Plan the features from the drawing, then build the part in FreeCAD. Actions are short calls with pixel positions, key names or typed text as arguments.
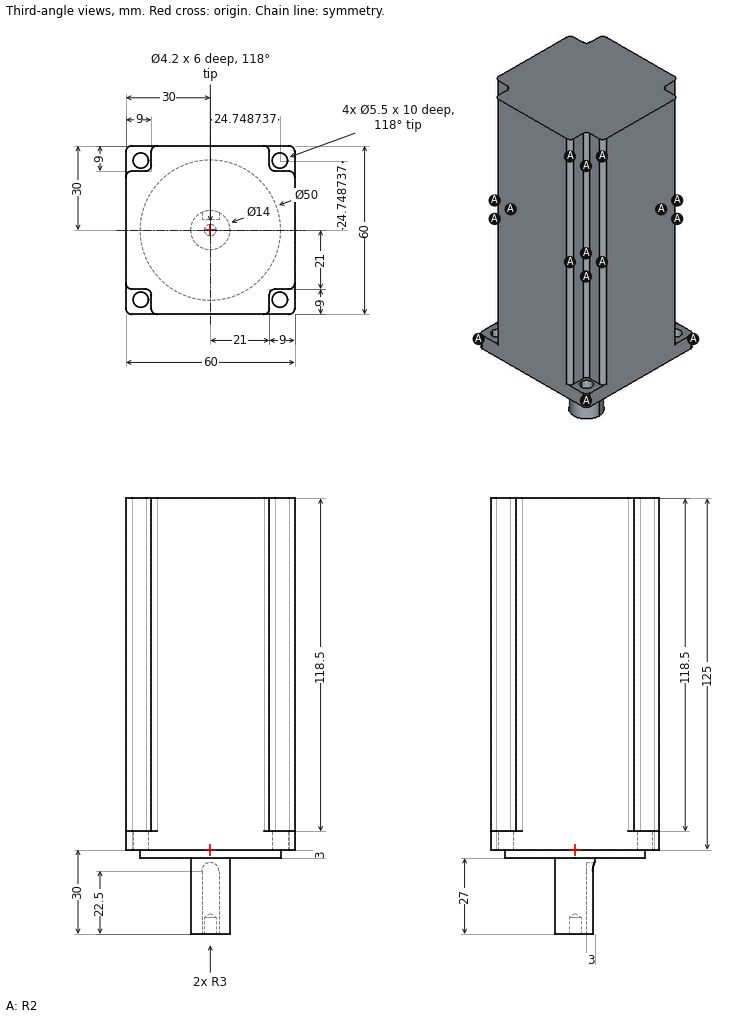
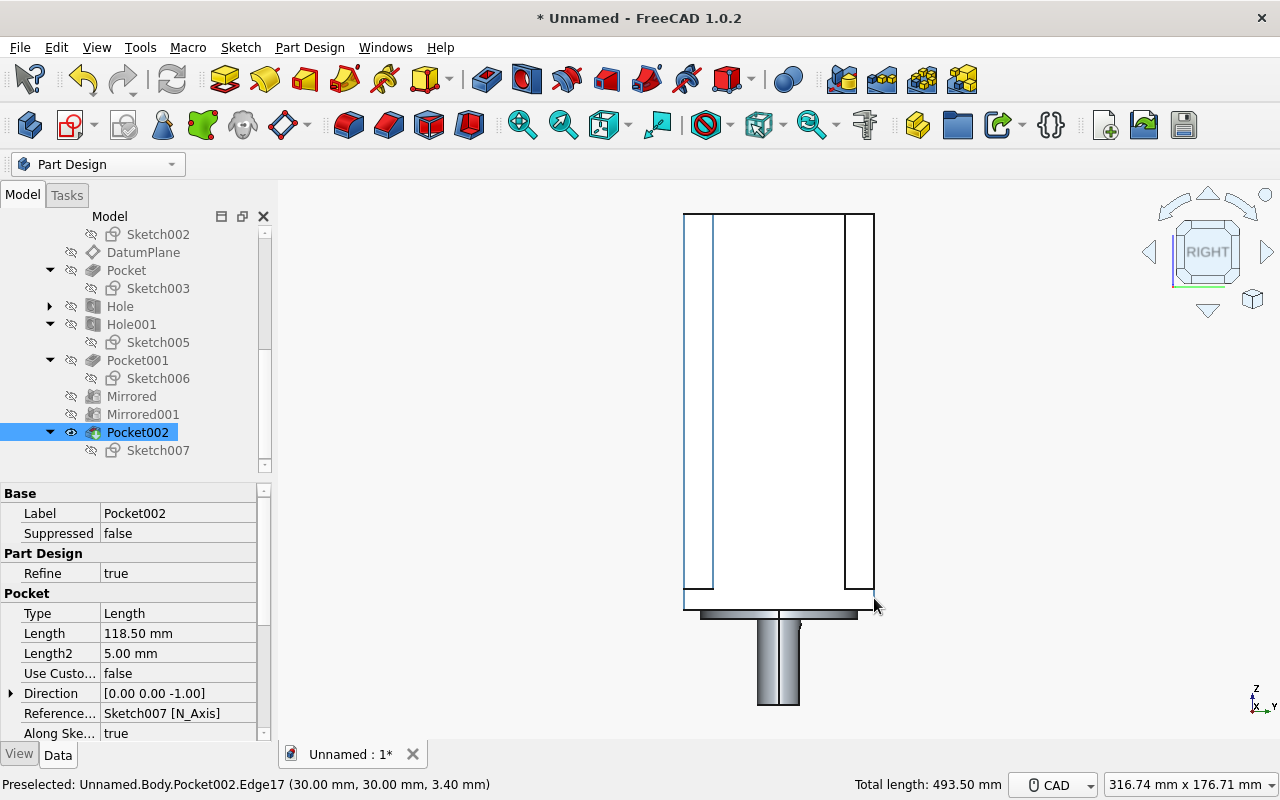
click(845, 401, ctrl)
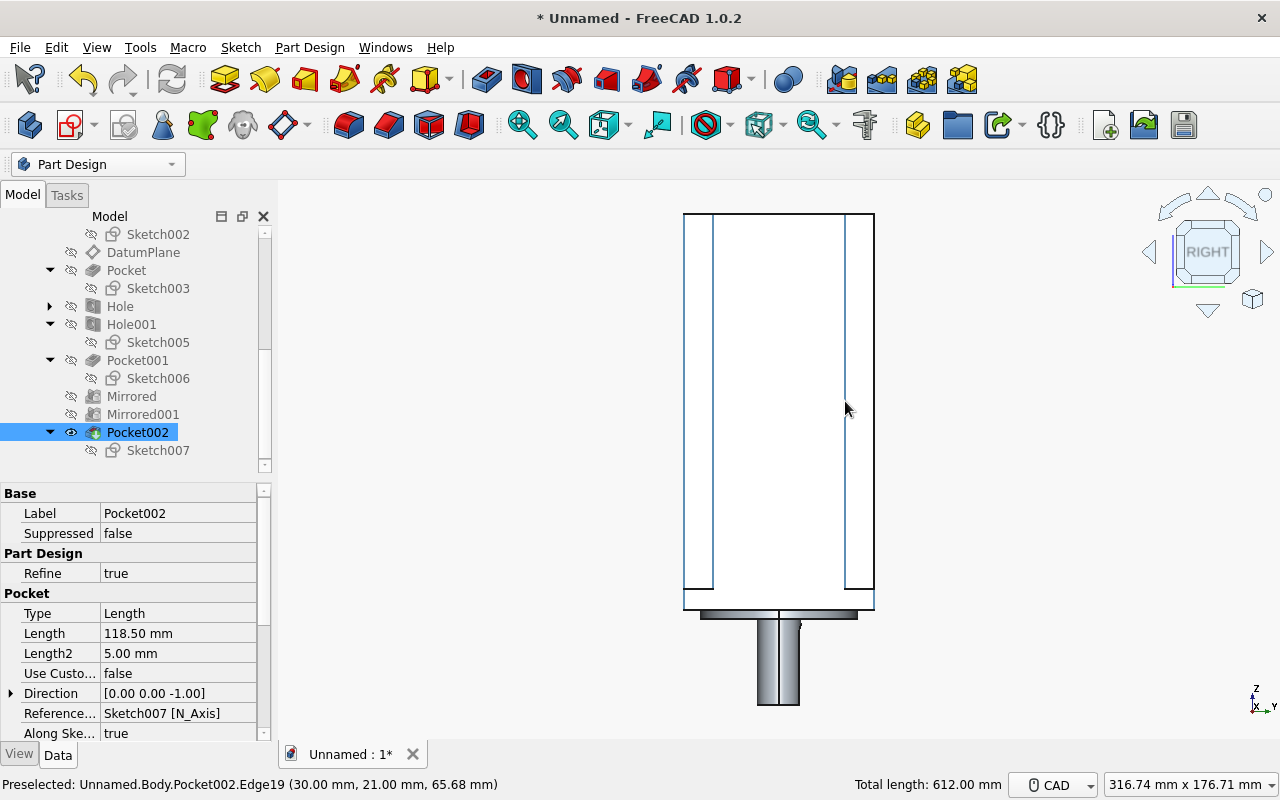
click(874, 401, ctrl)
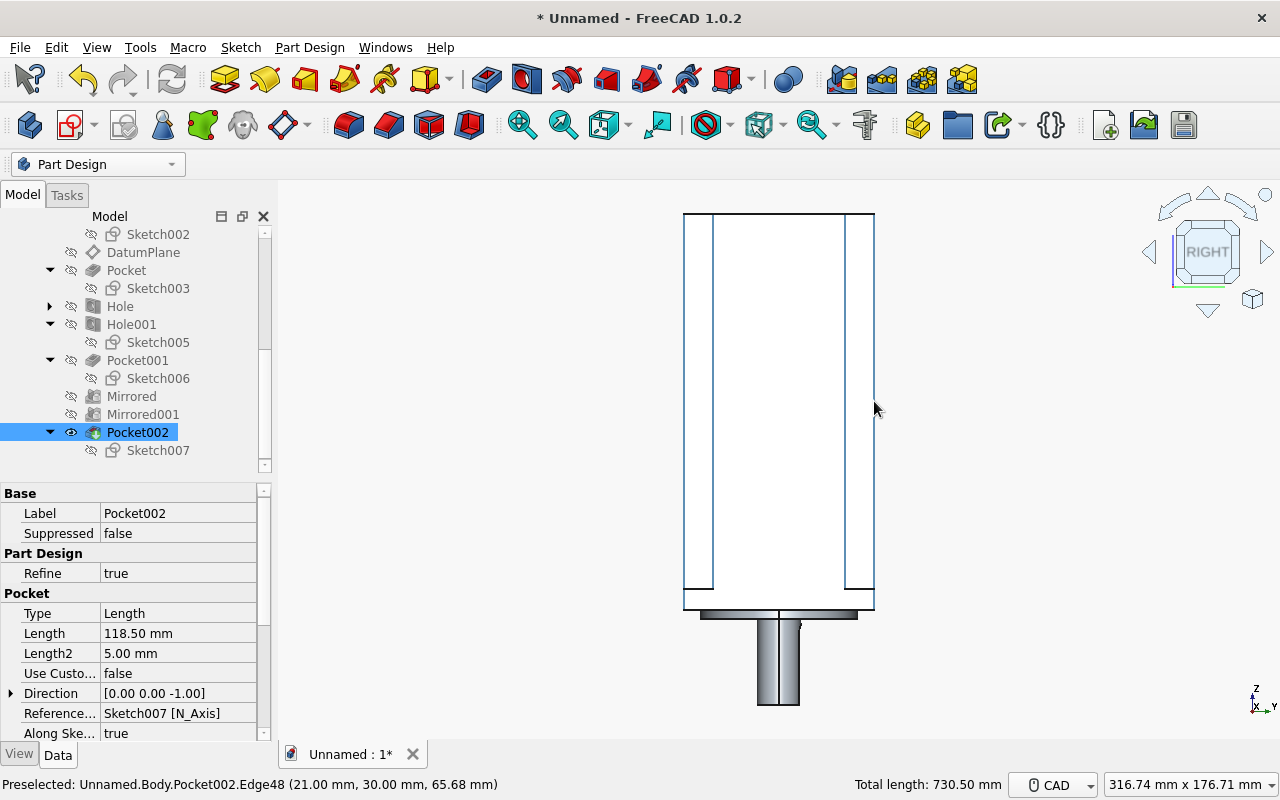
key(5)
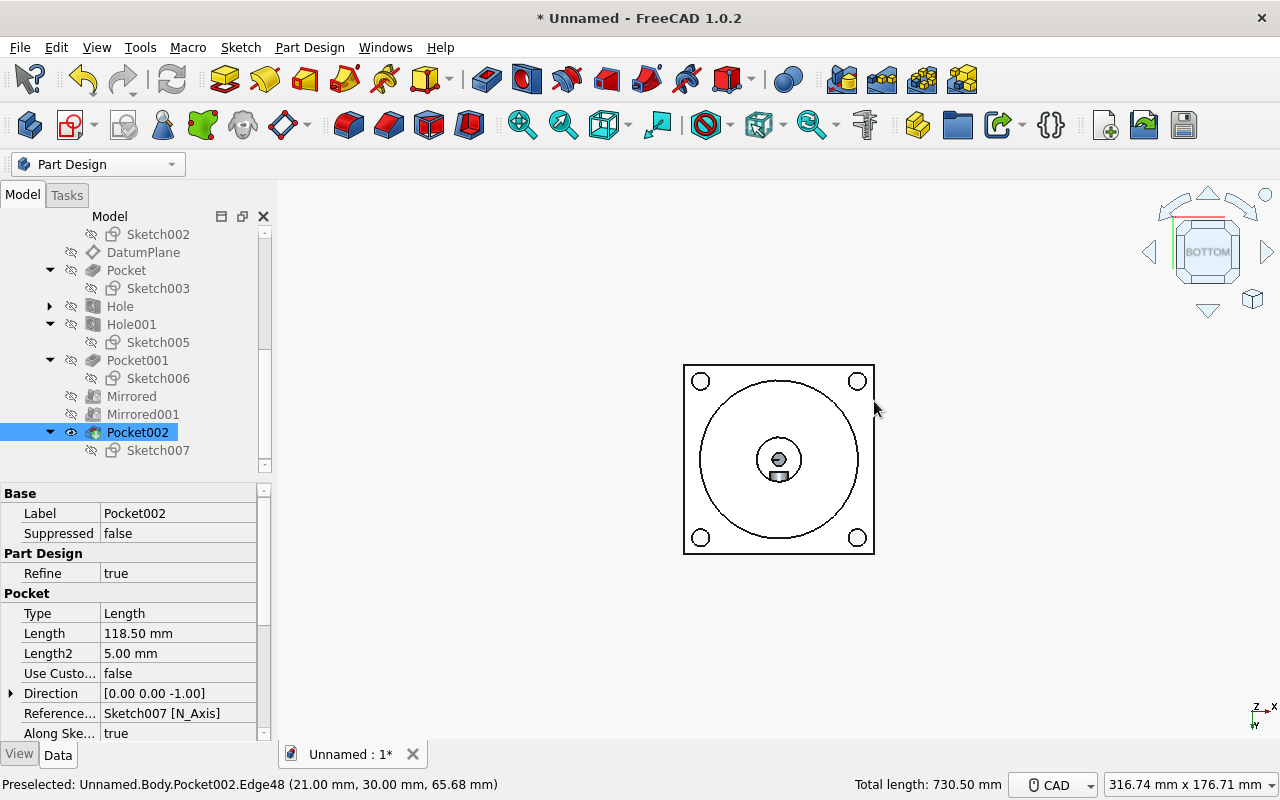
click(524, 126)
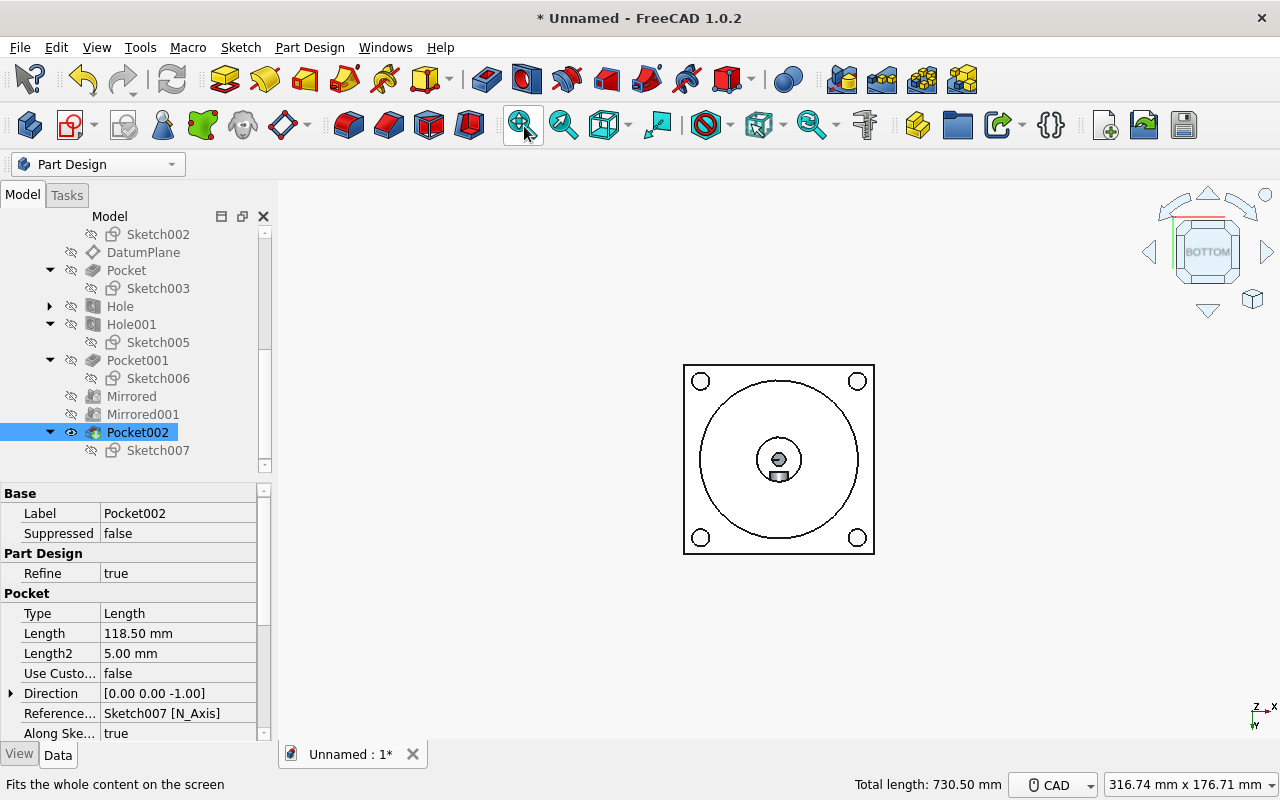
key(4)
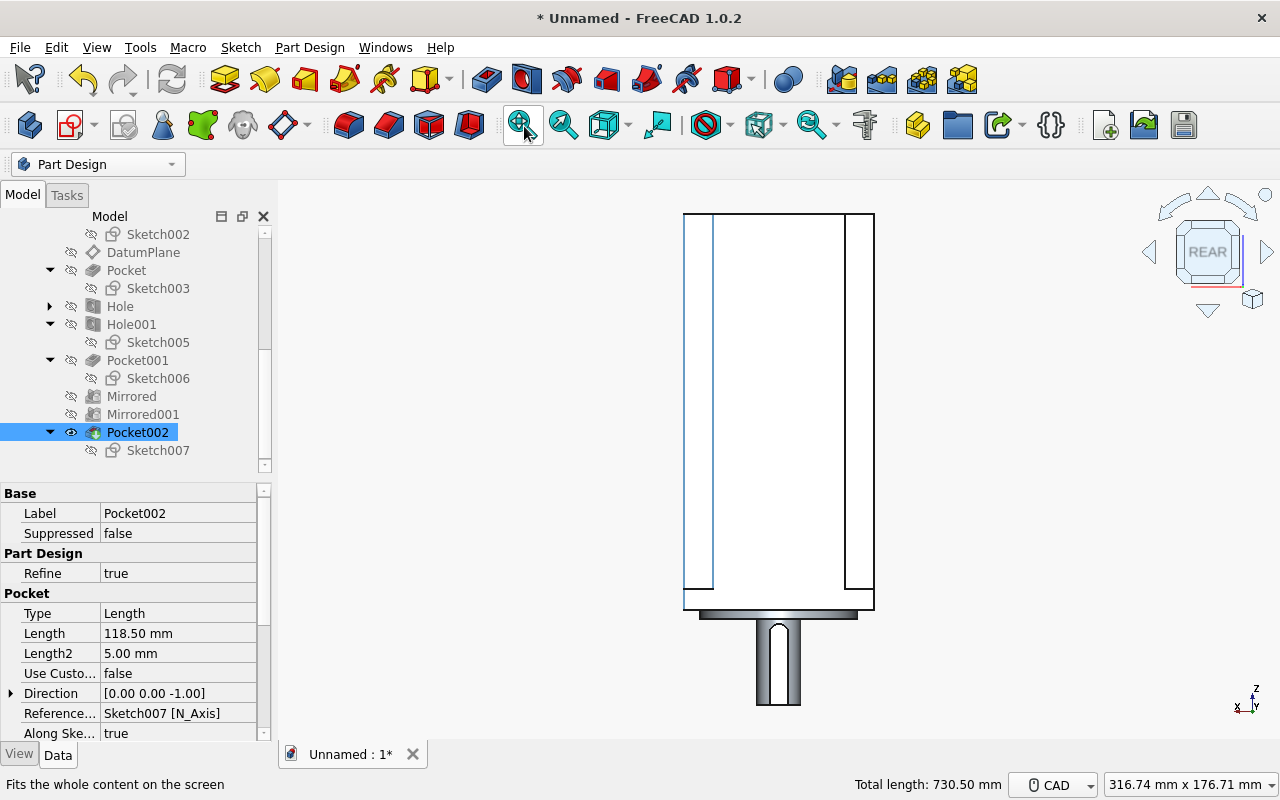
click(874, 598, ctrl)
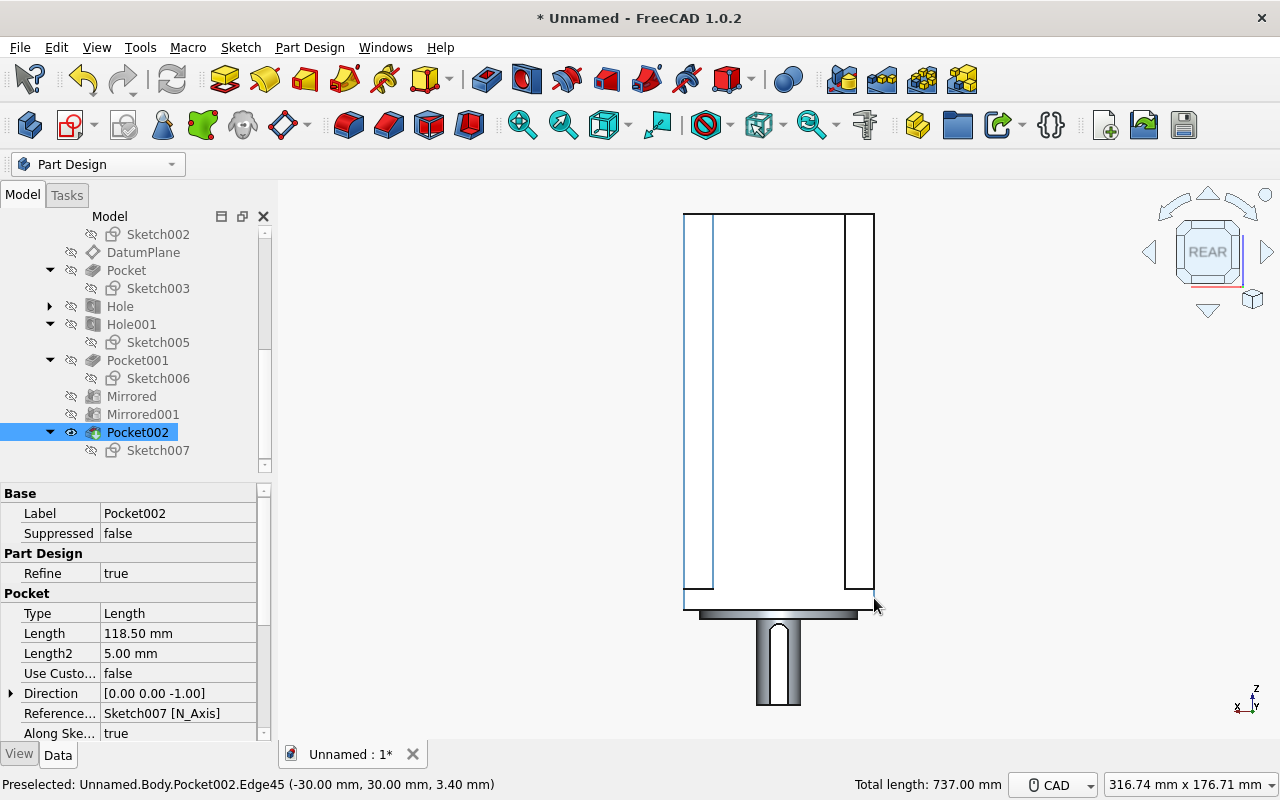
click(874, 401, ctrl)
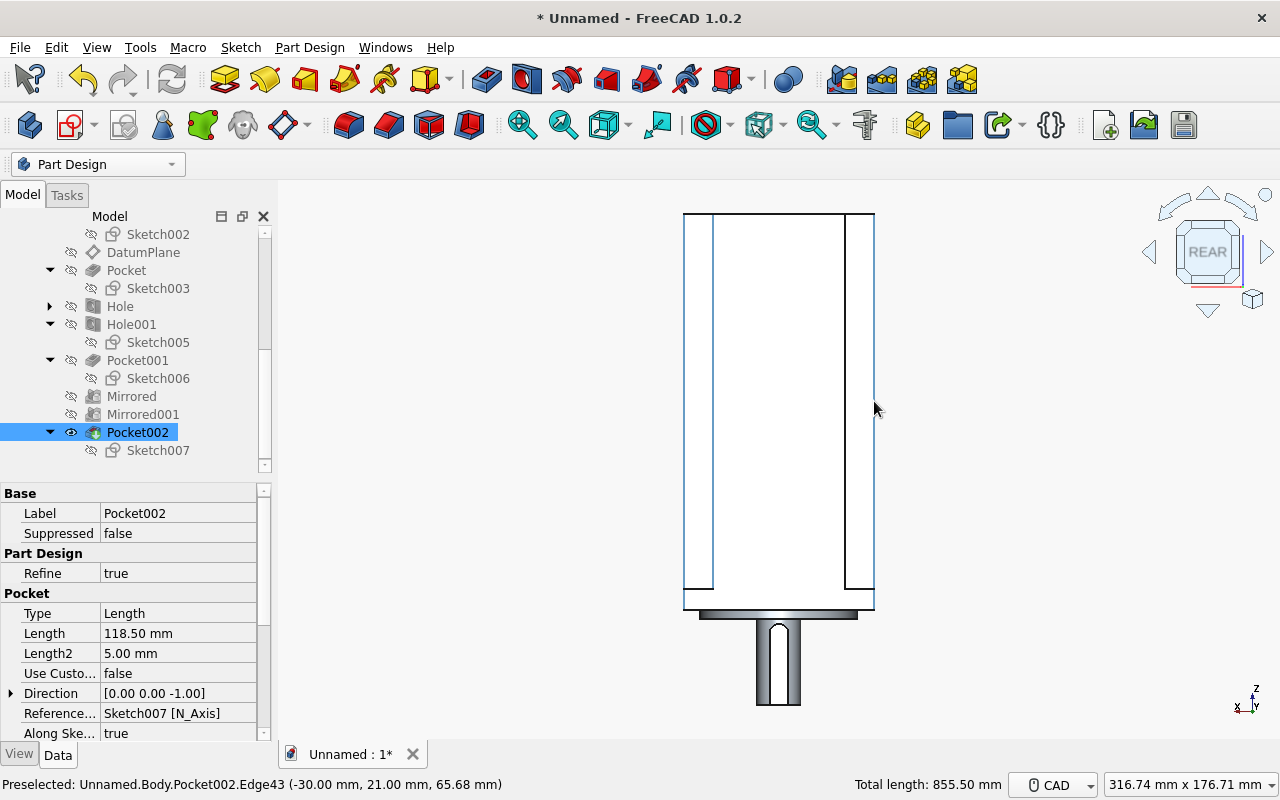
click(845, 401, ctrl)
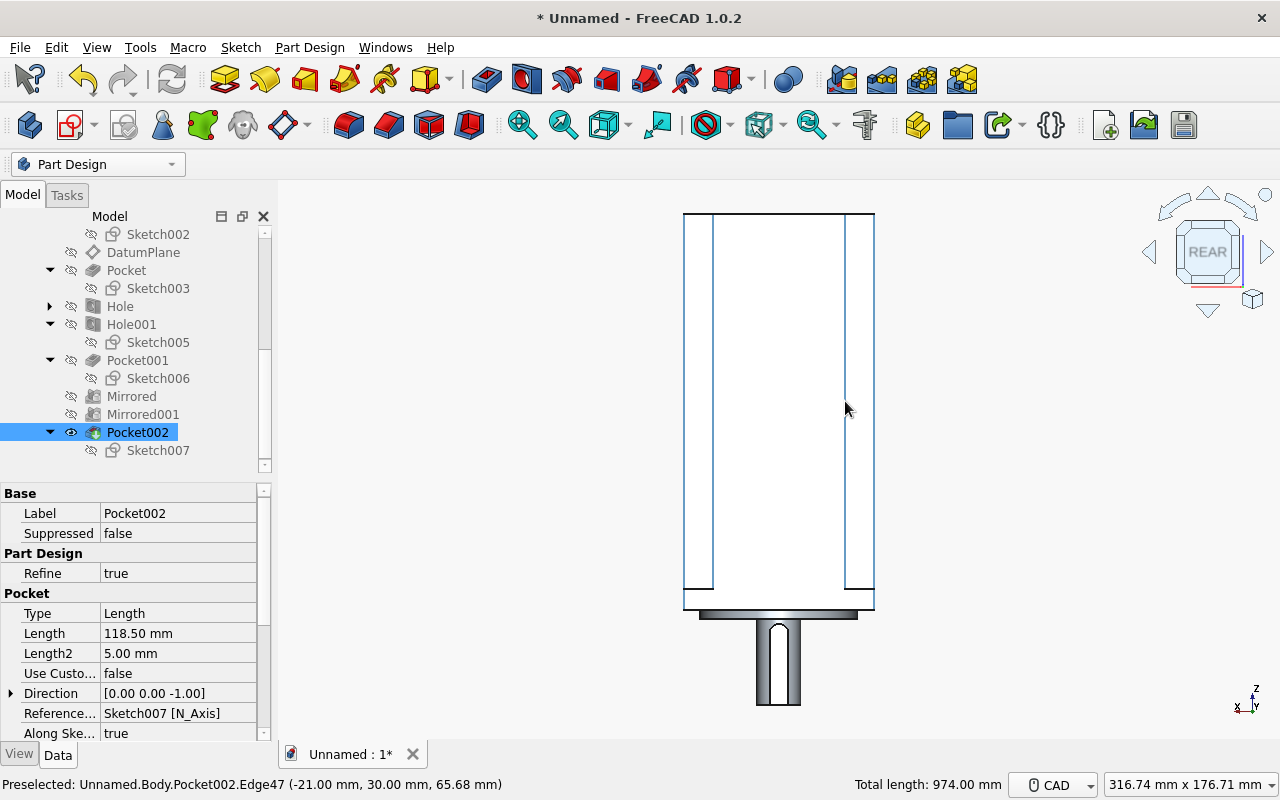
key(6)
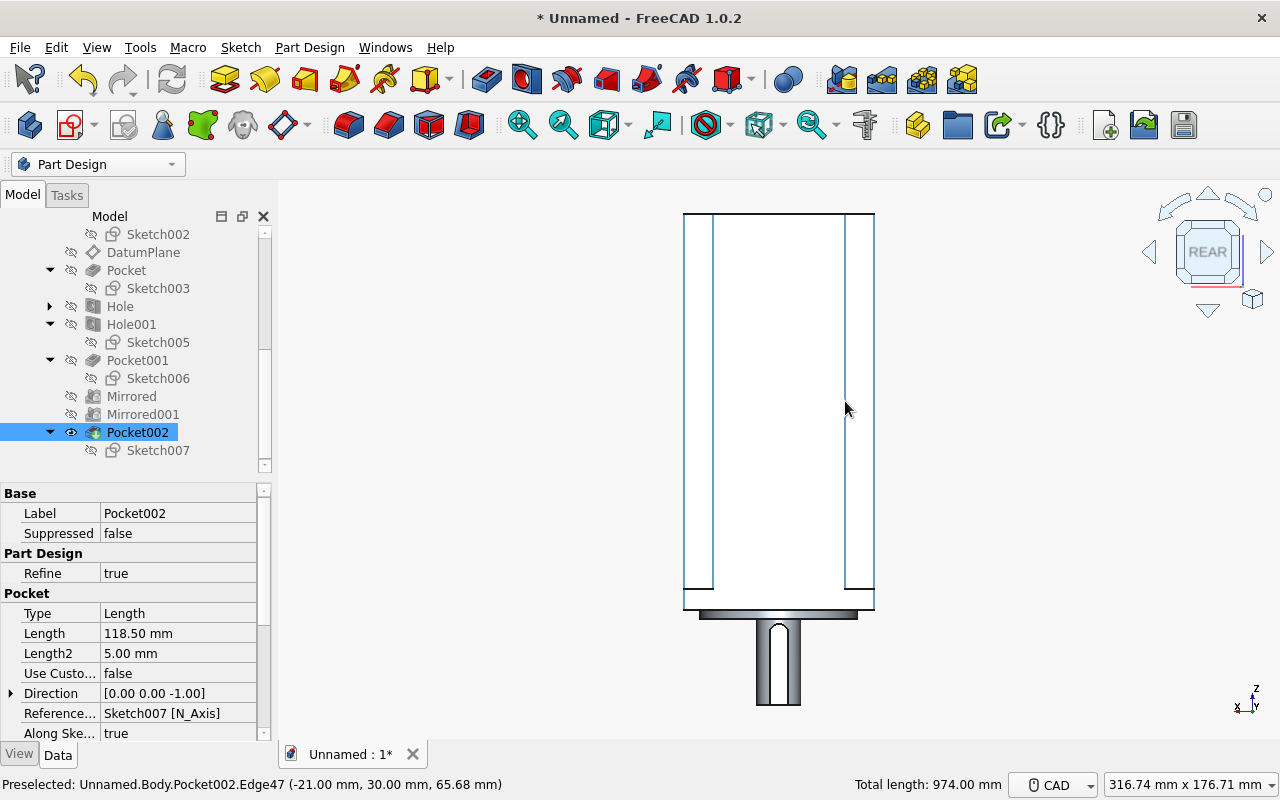
key(v)
key(3)